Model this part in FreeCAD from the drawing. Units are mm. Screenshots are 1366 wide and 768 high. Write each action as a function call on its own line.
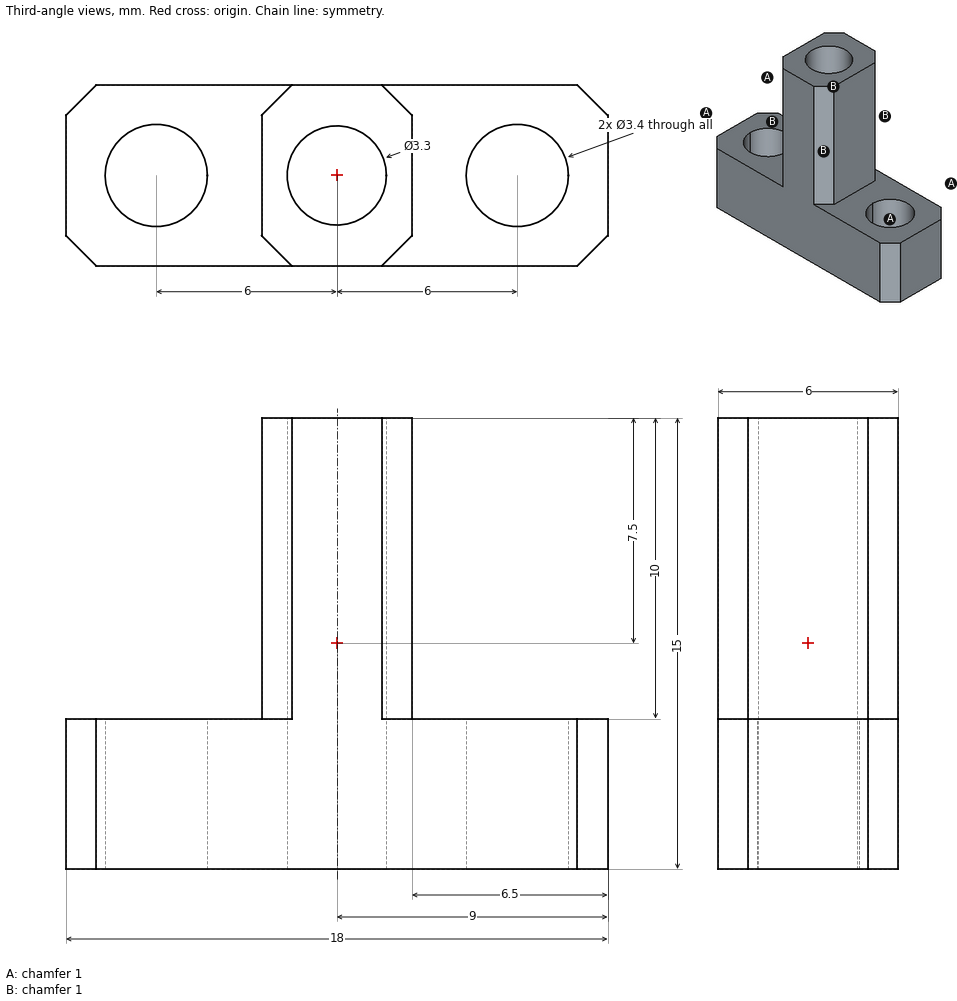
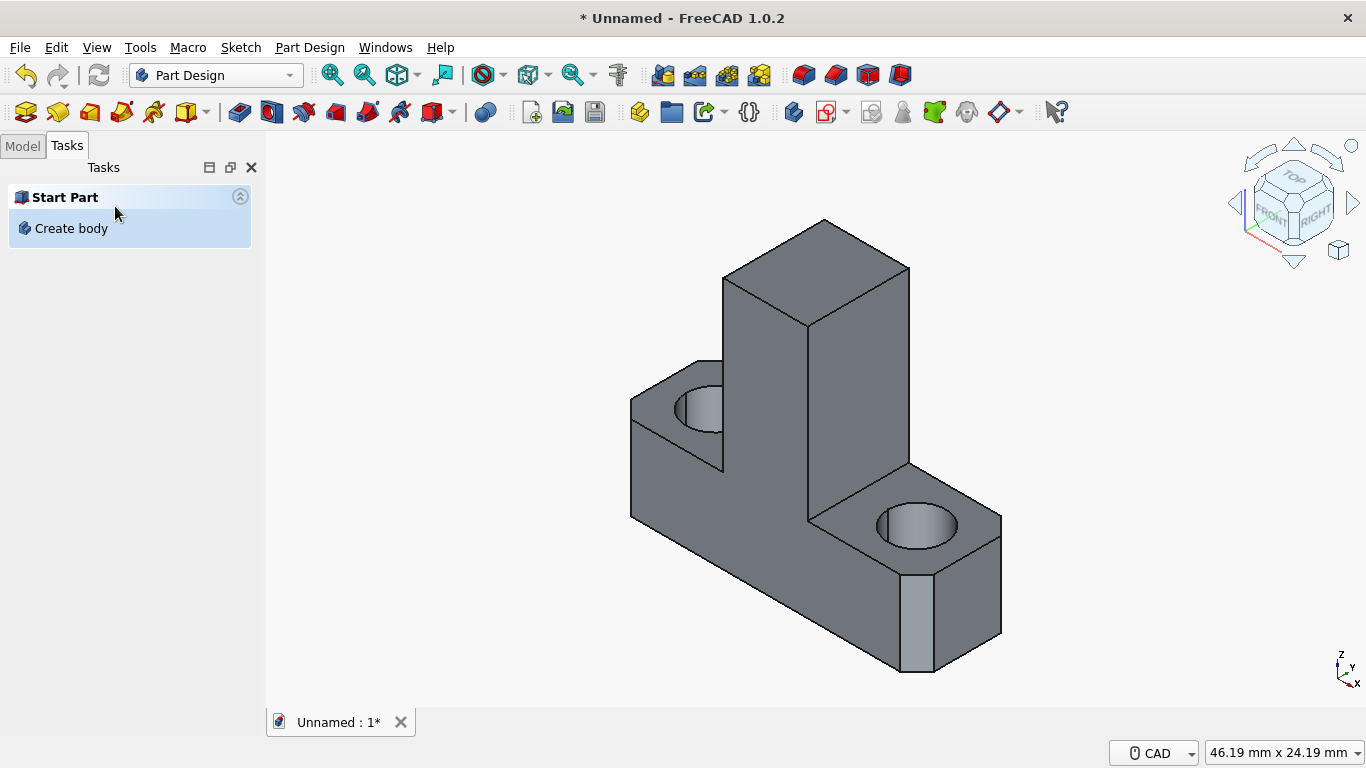
key(5)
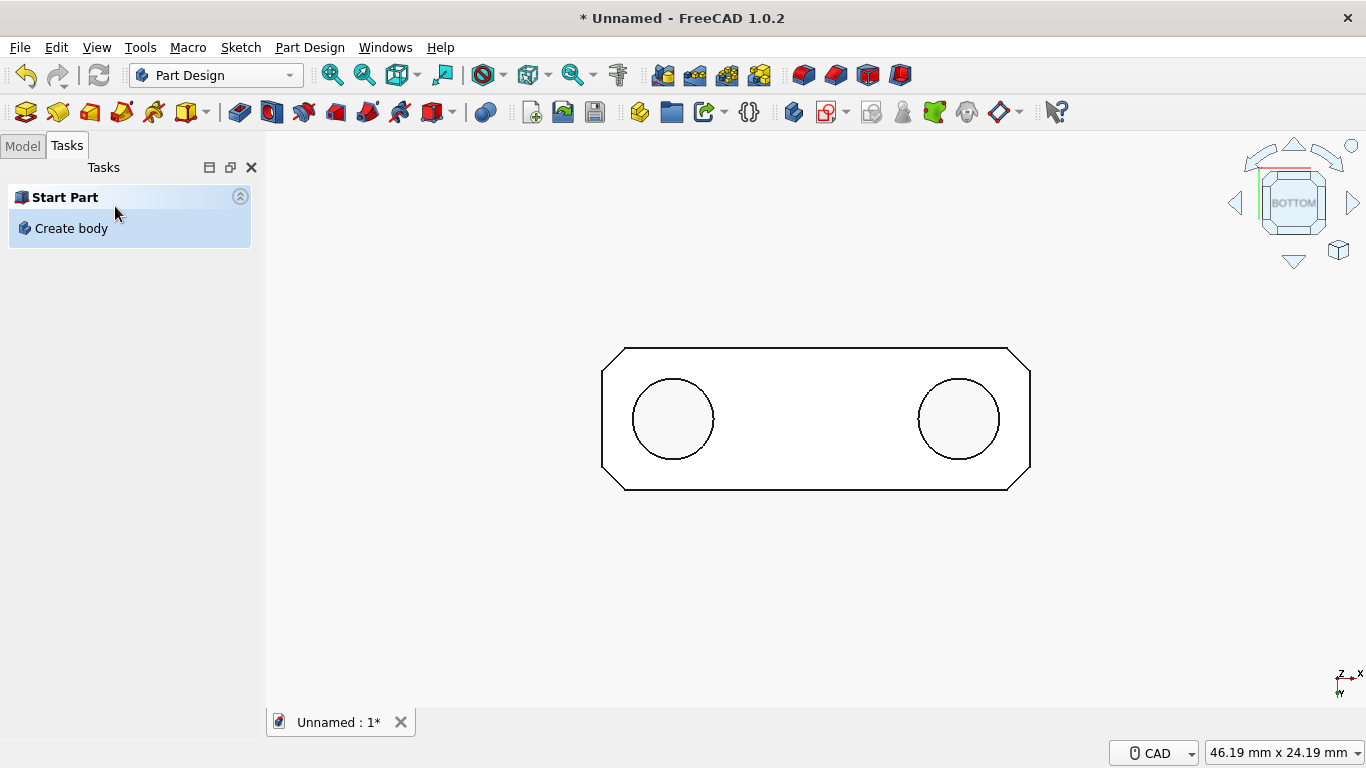
click(334, 76)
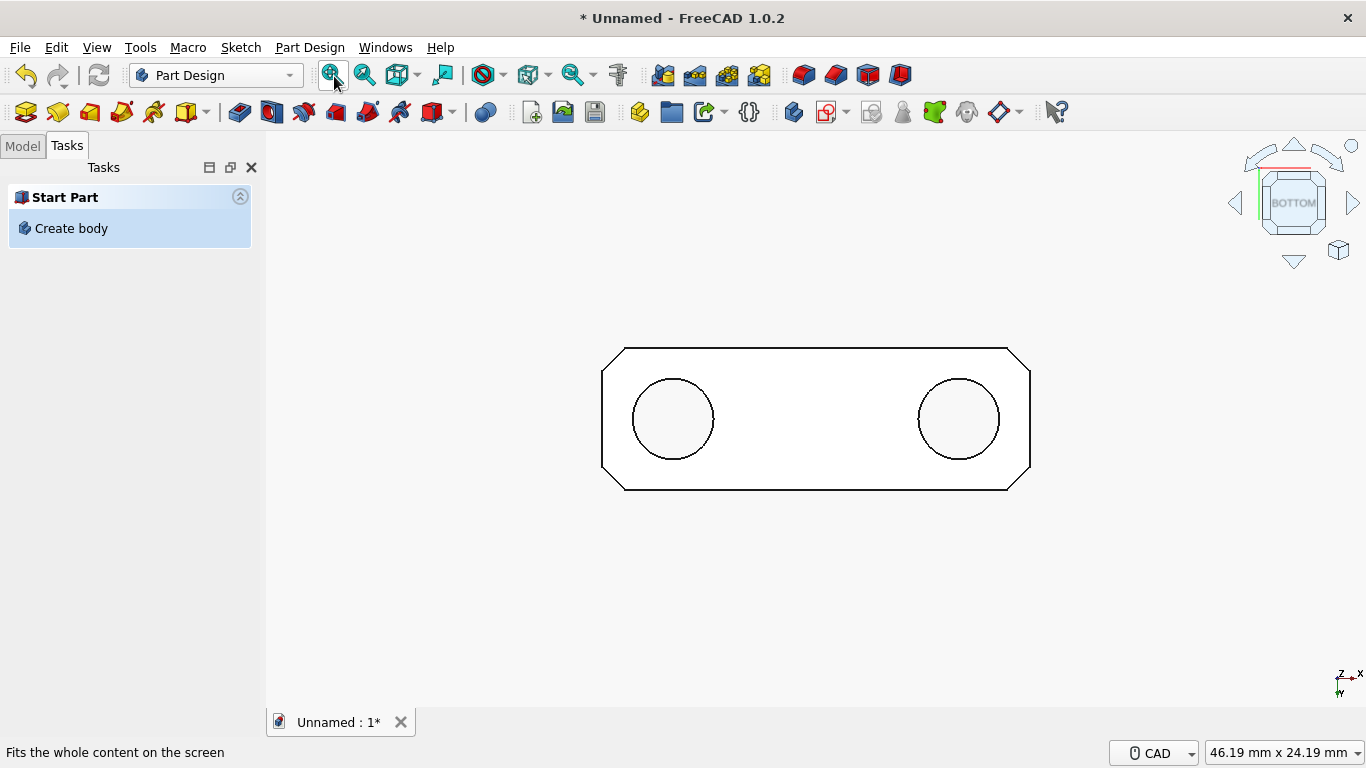
click(816, 418)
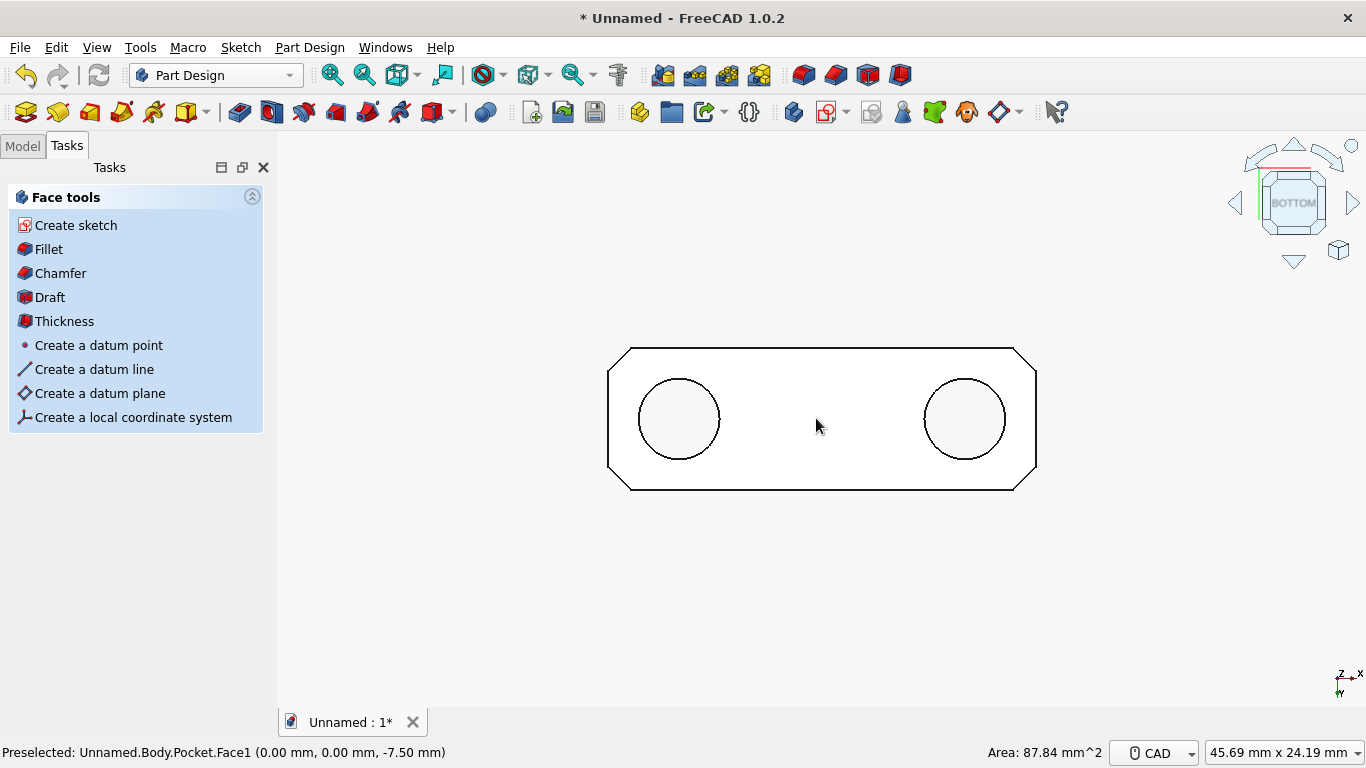
click(826, 112)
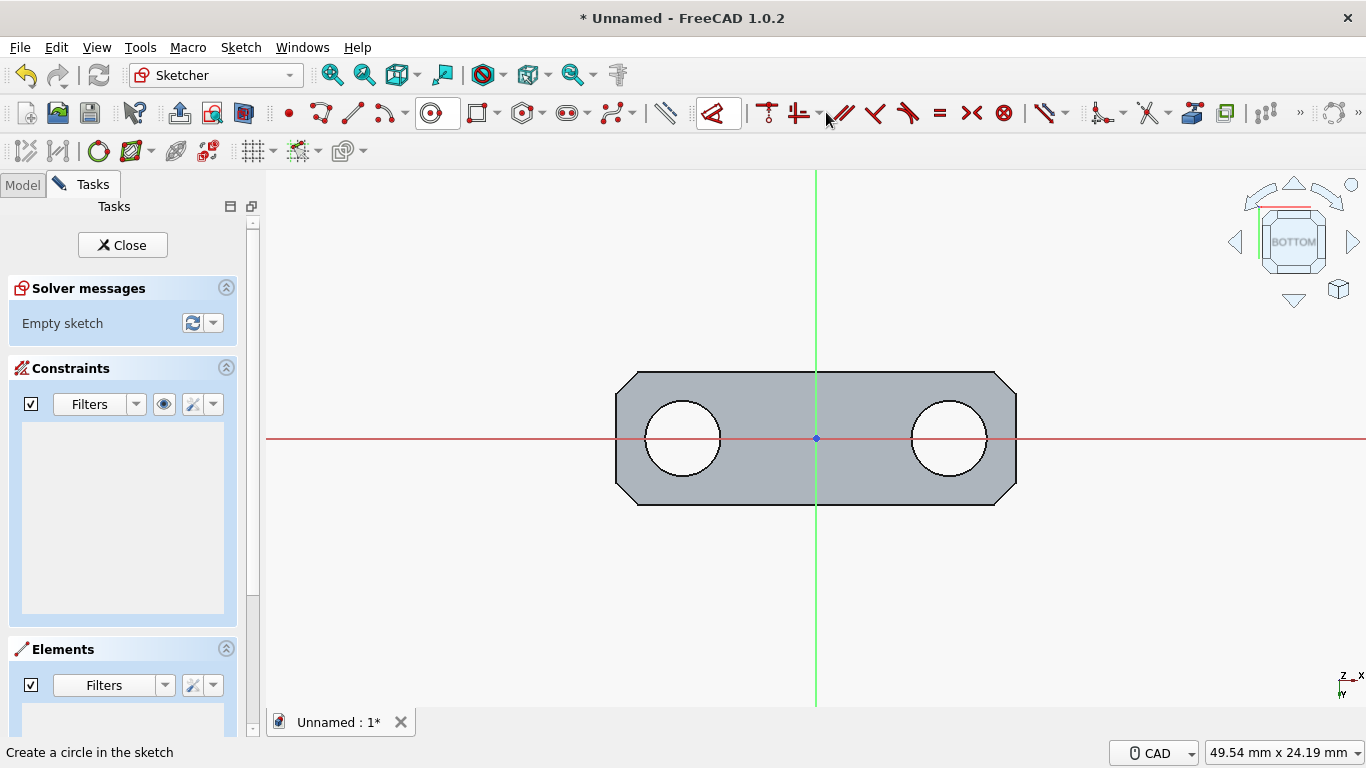
scroll(833, 438, up, 8)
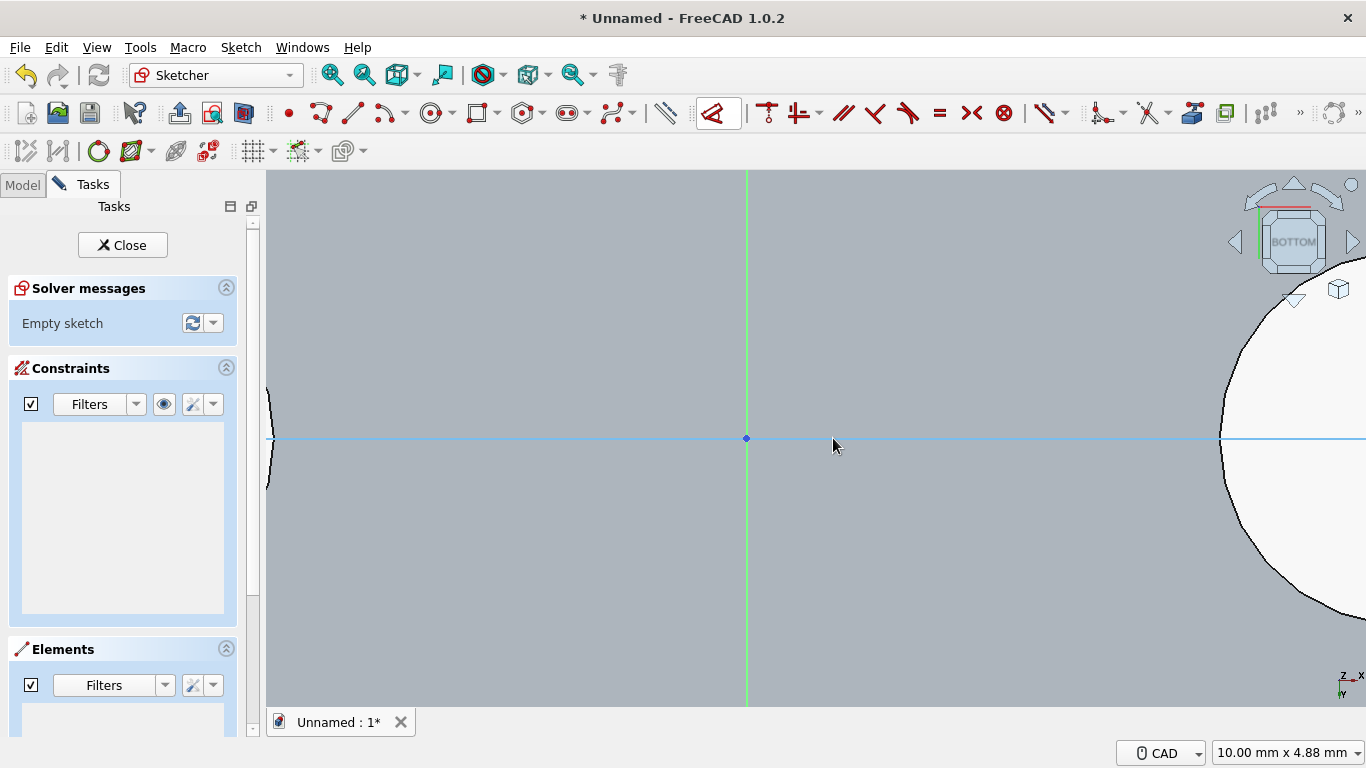
click(432, 114)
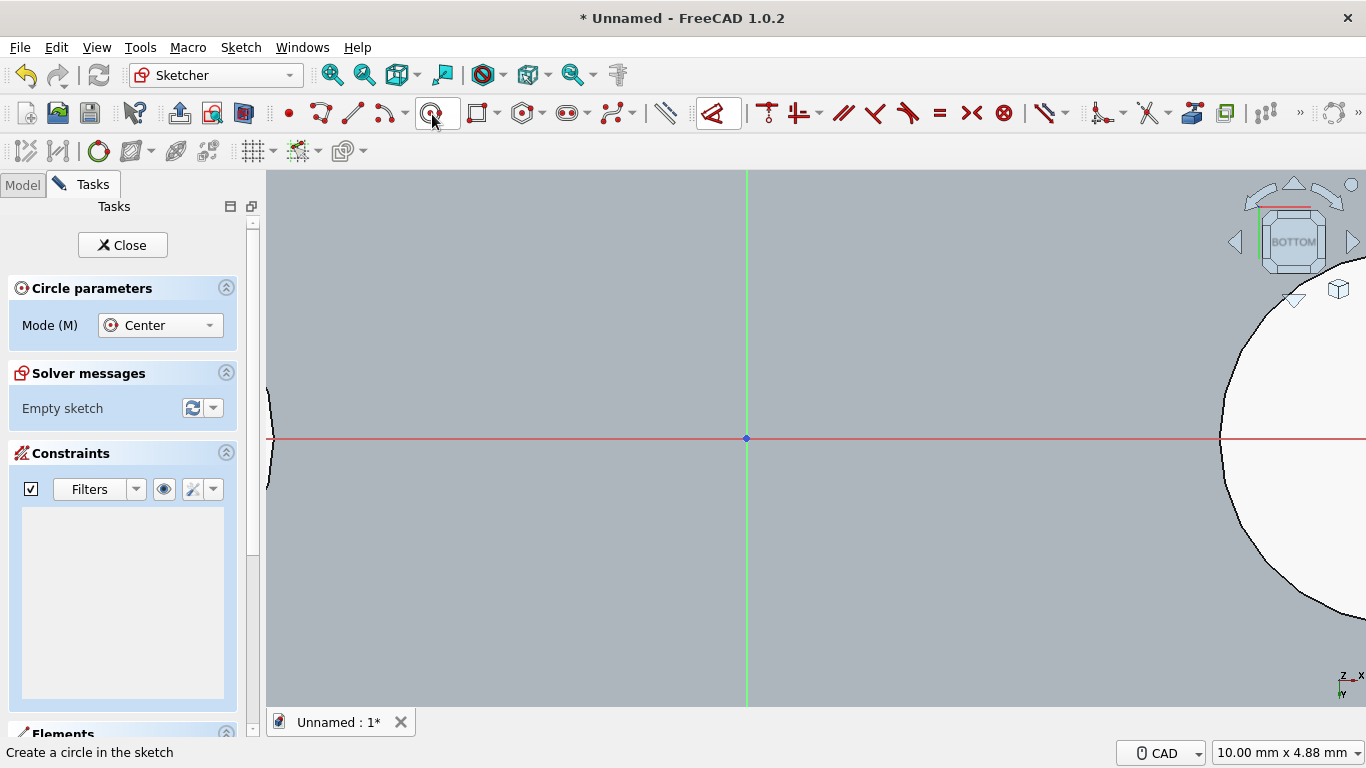
click(747, 438)
click(875, 310)
key(Escape)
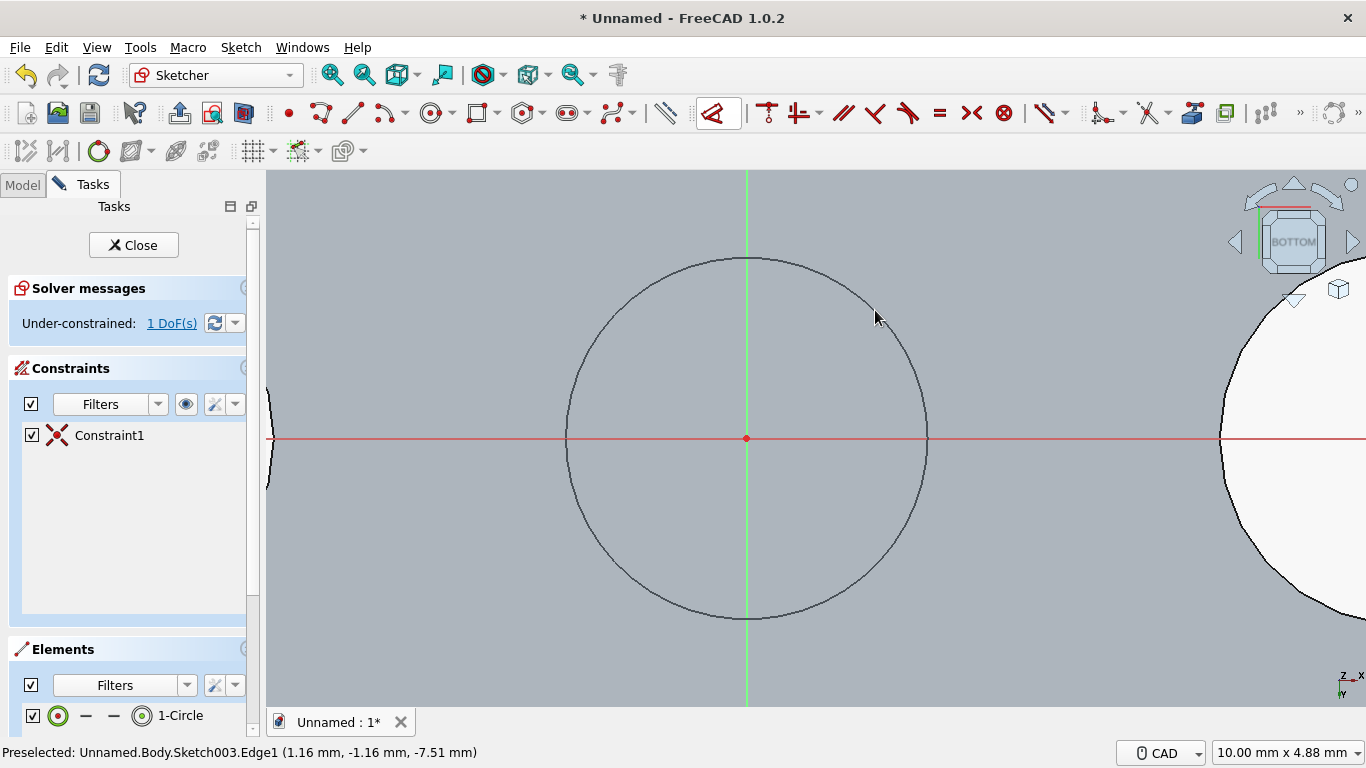
click(874, 310)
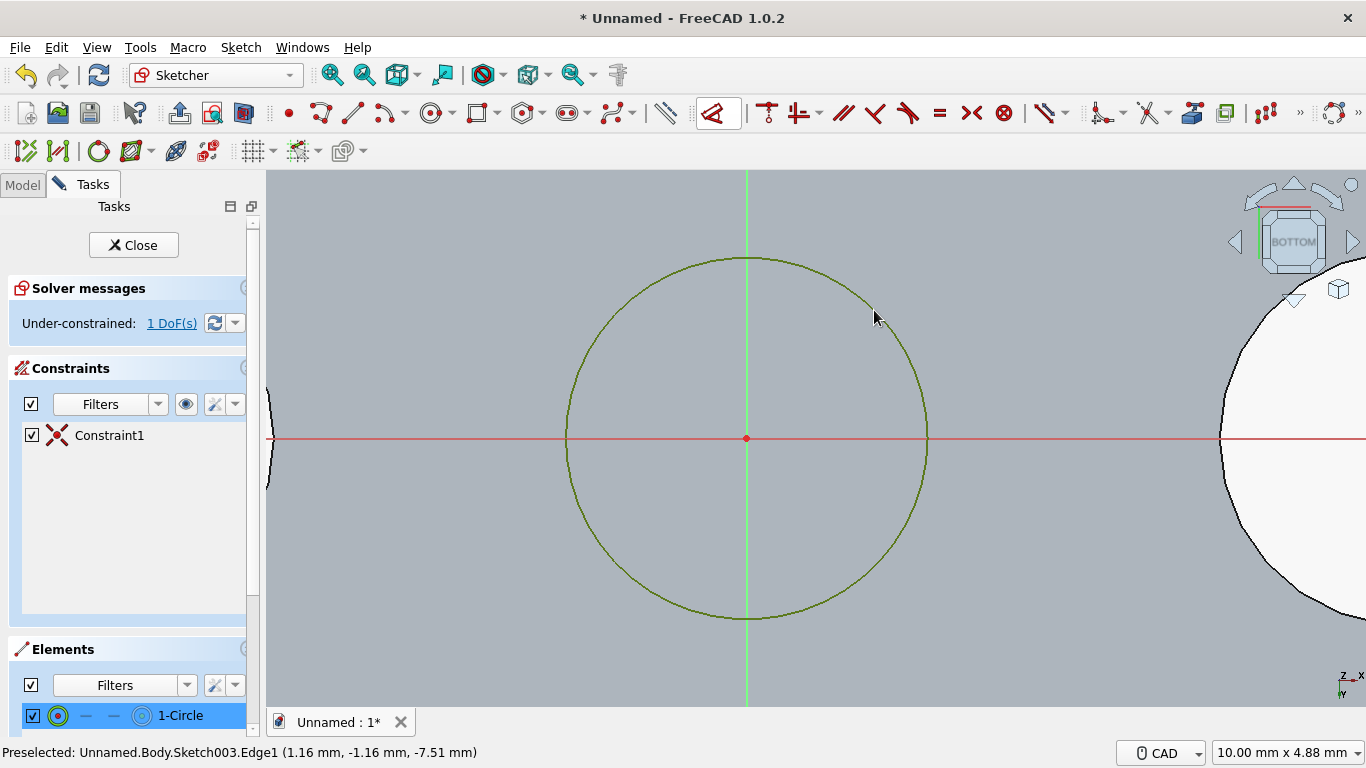
click(736, 114)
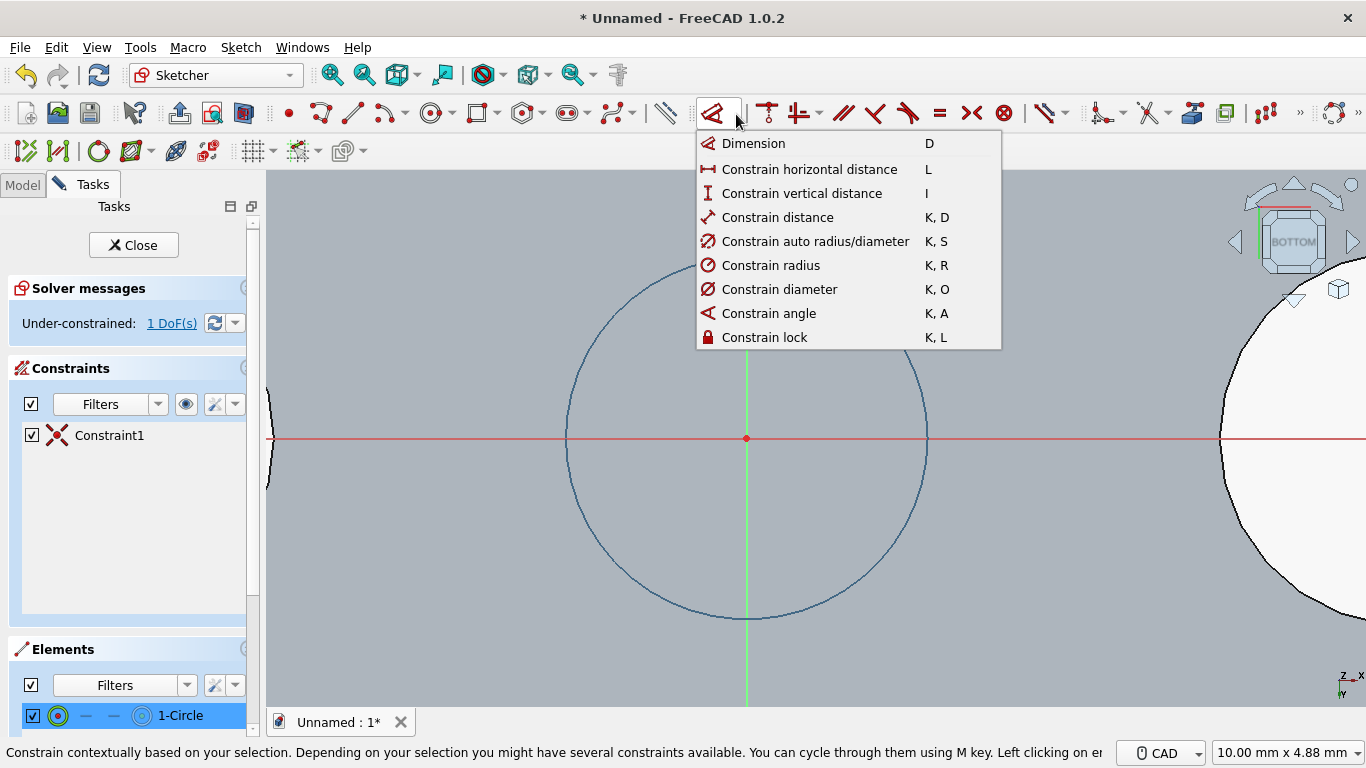
click(849, 289)